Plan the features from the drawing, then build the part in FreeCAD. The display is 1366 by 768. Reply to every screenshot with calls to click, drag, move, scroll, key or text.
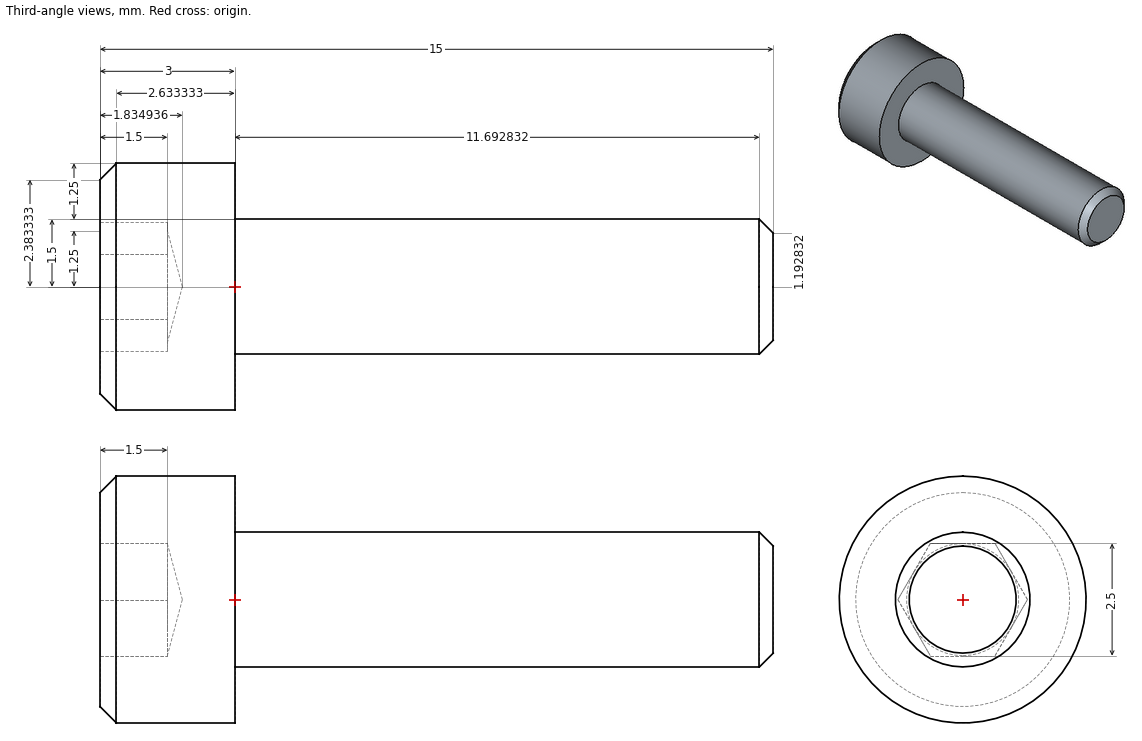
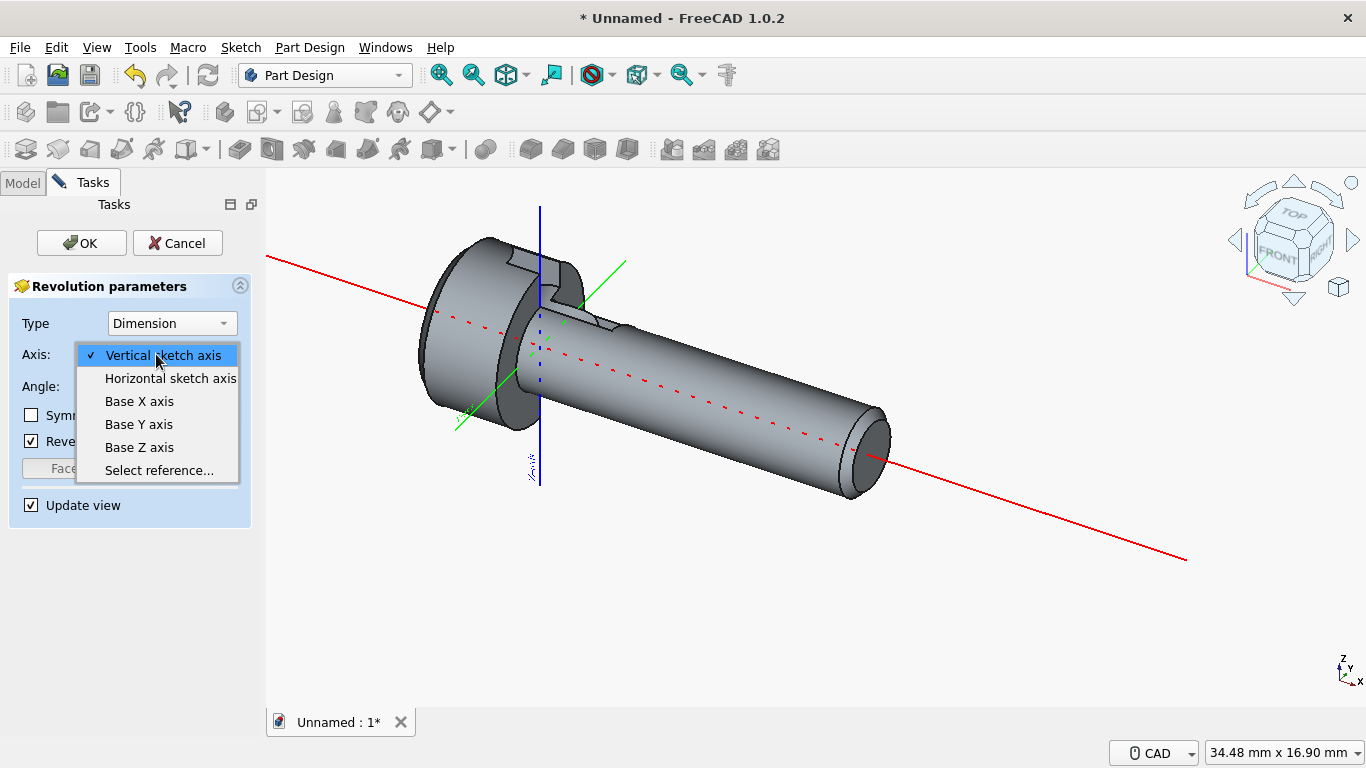
click(156, 378)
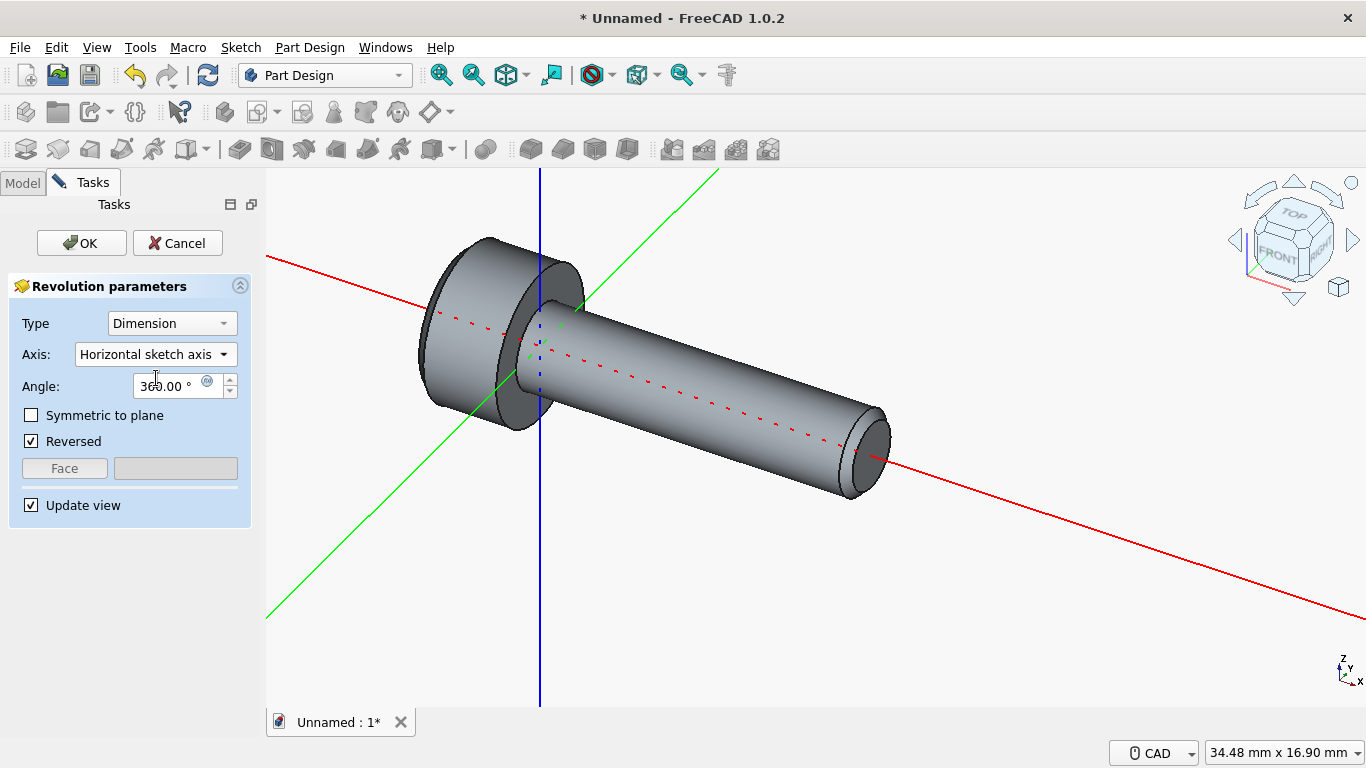
click(82, 243)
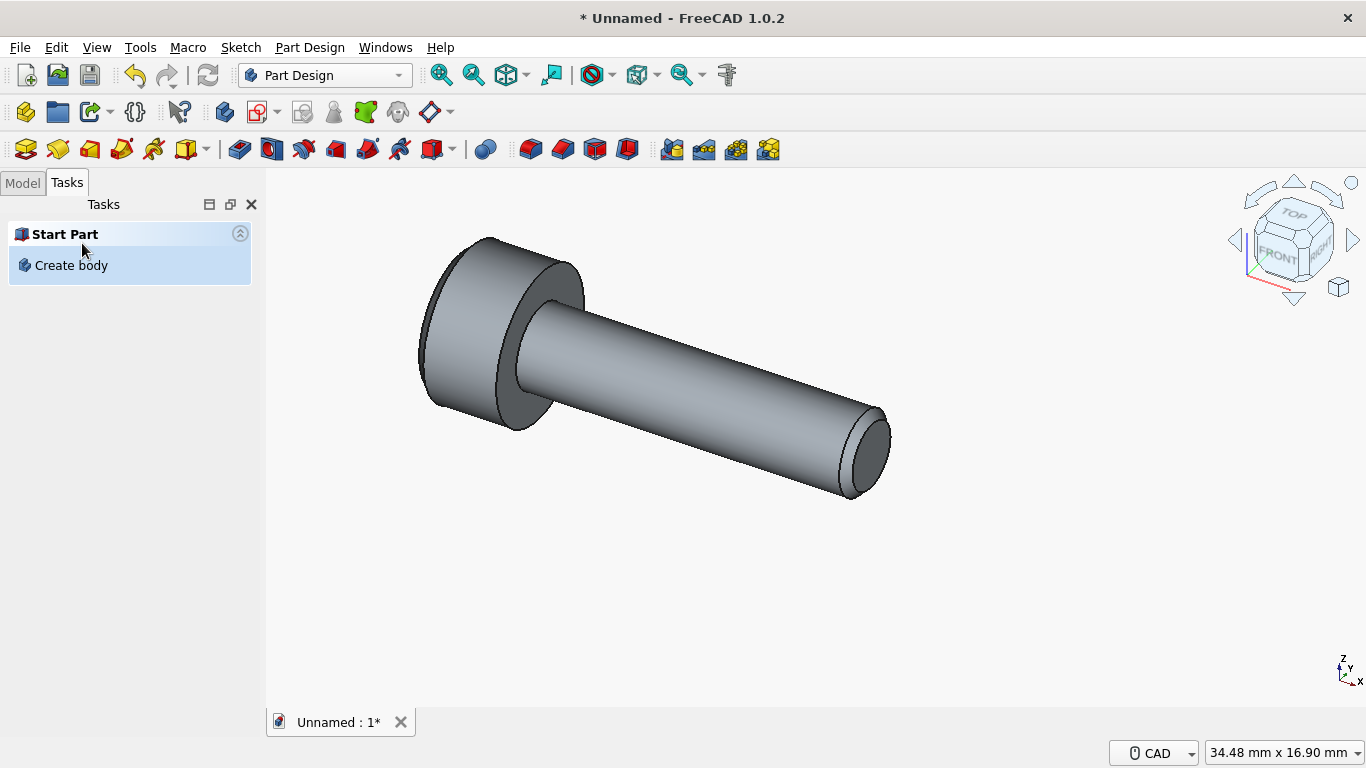
key(6)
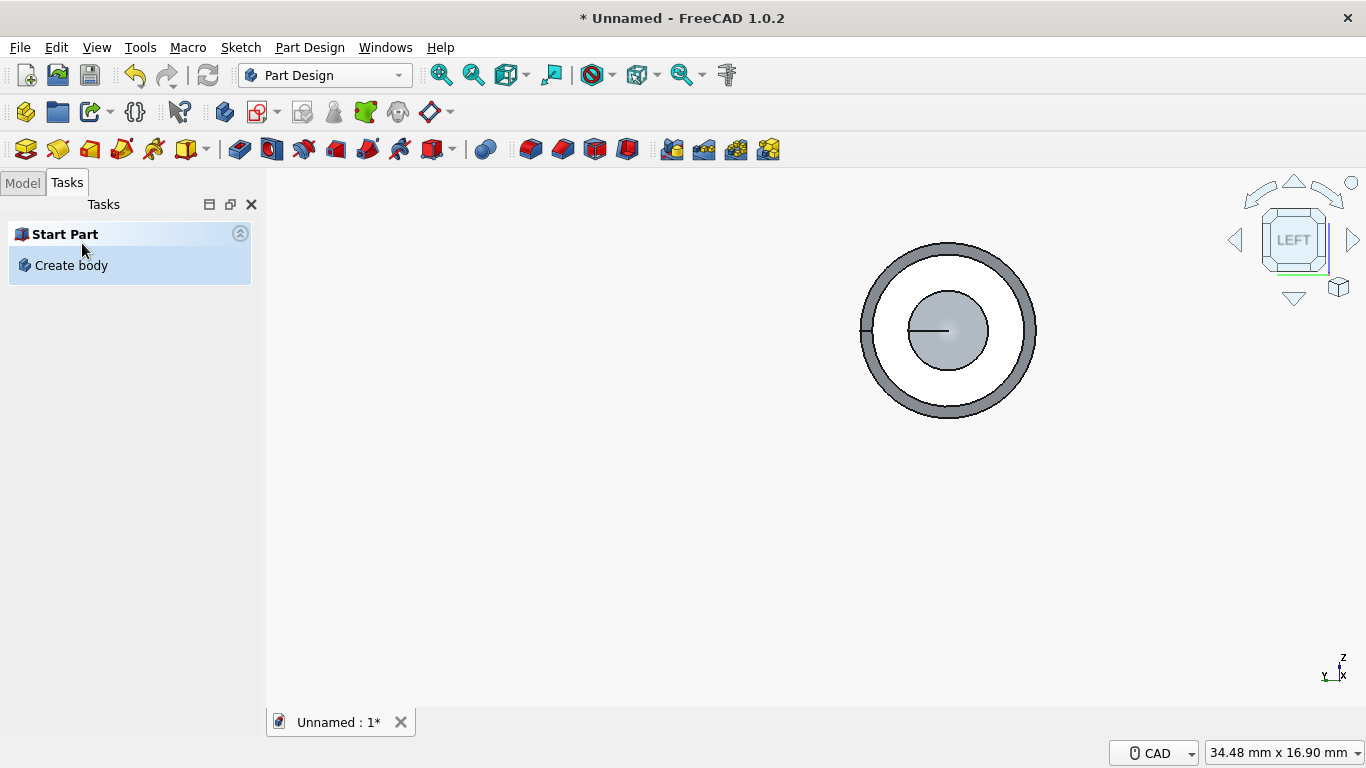
click(442, 76)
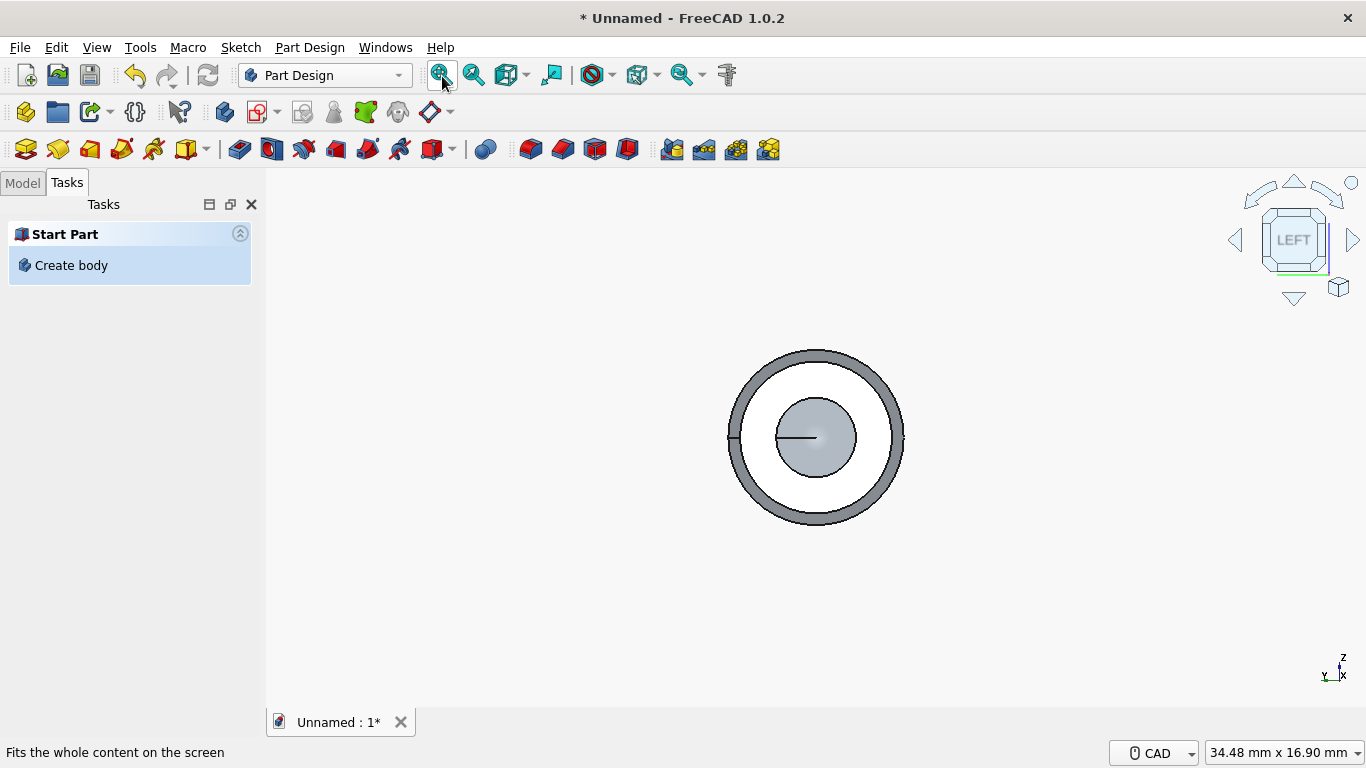
click(859, 480)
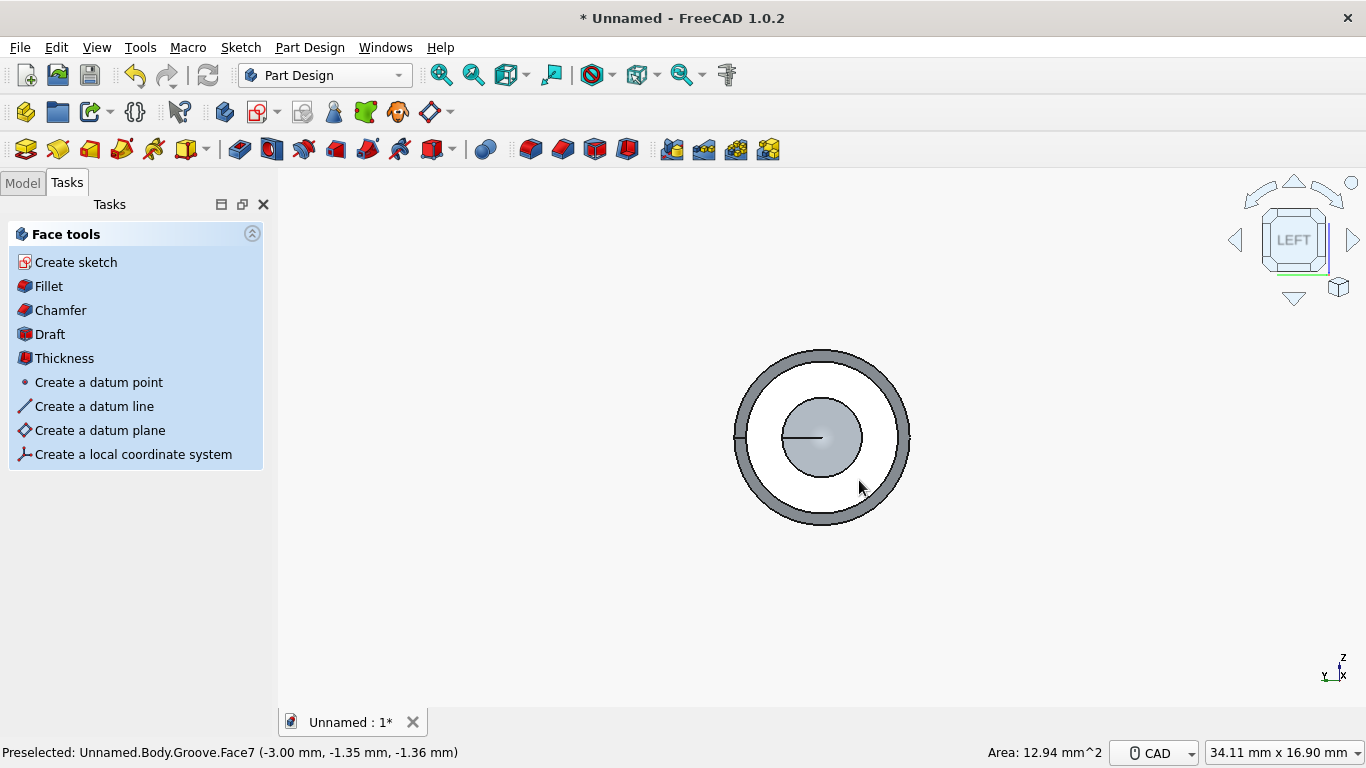
click(258, 112)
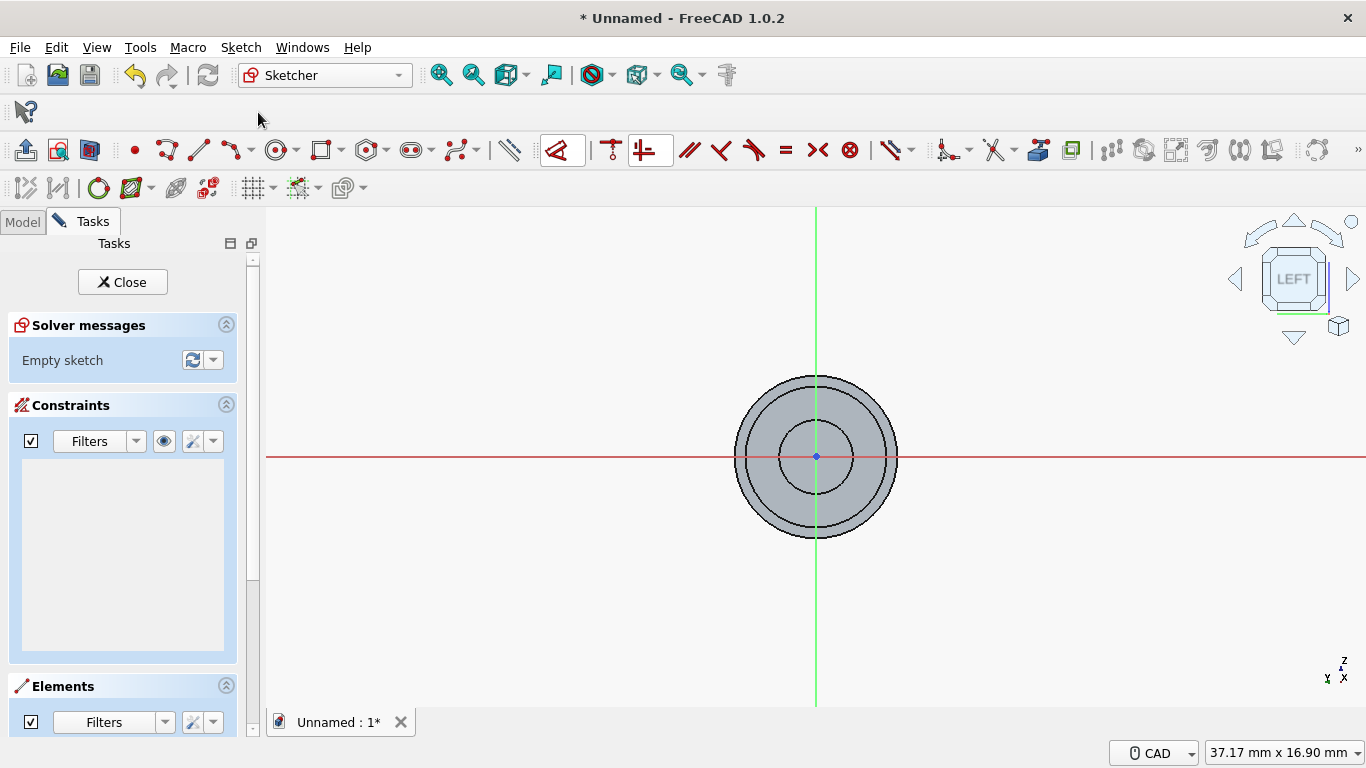
scroll(838, 457, up, 7)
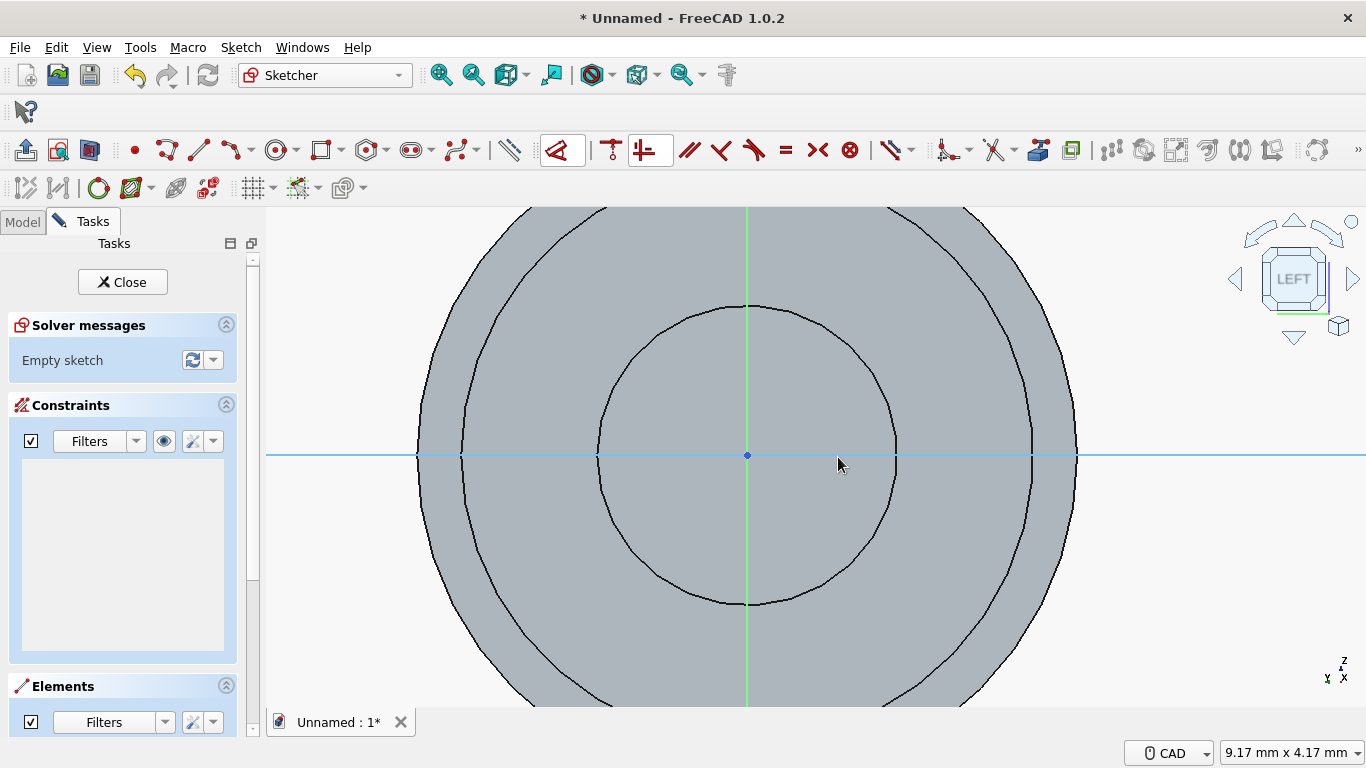
click(366, 150)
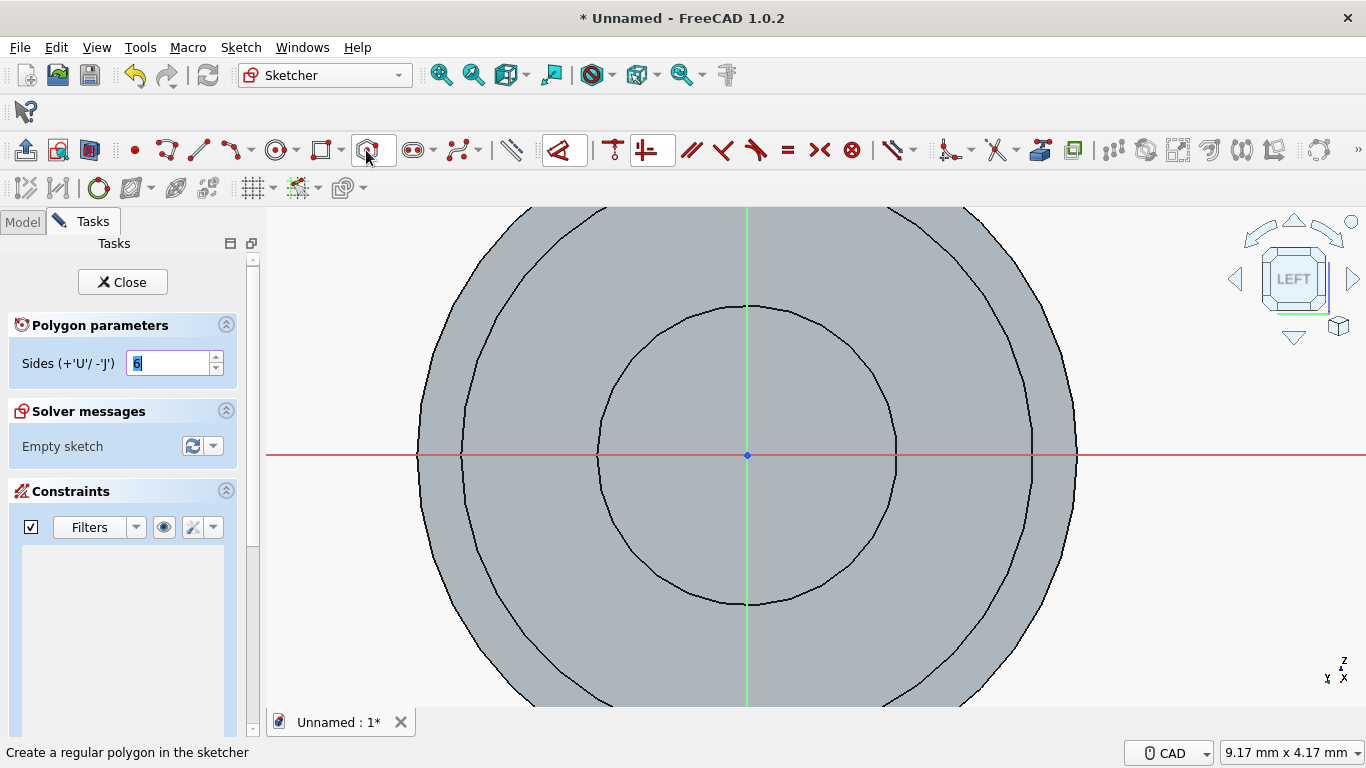
click(747, 455)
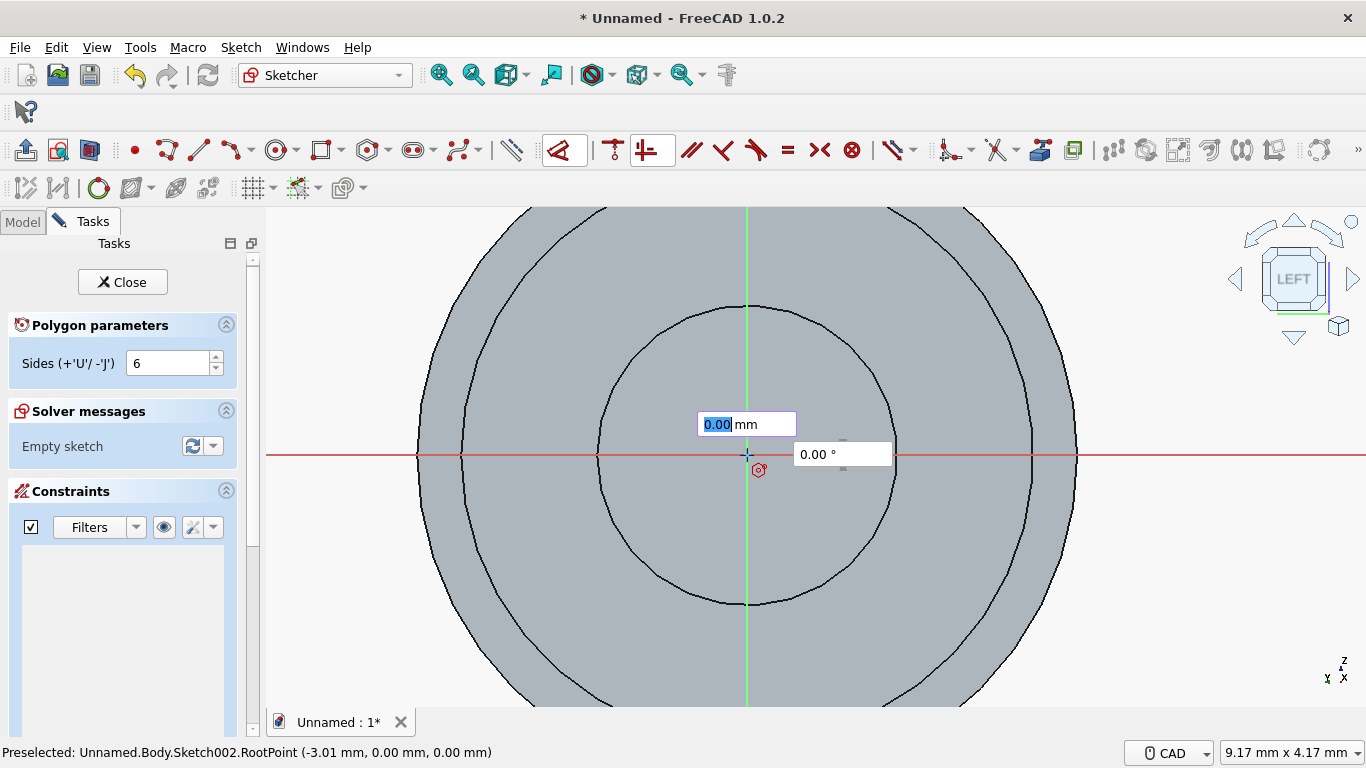
click(920, 455)
right_click(920, 455)